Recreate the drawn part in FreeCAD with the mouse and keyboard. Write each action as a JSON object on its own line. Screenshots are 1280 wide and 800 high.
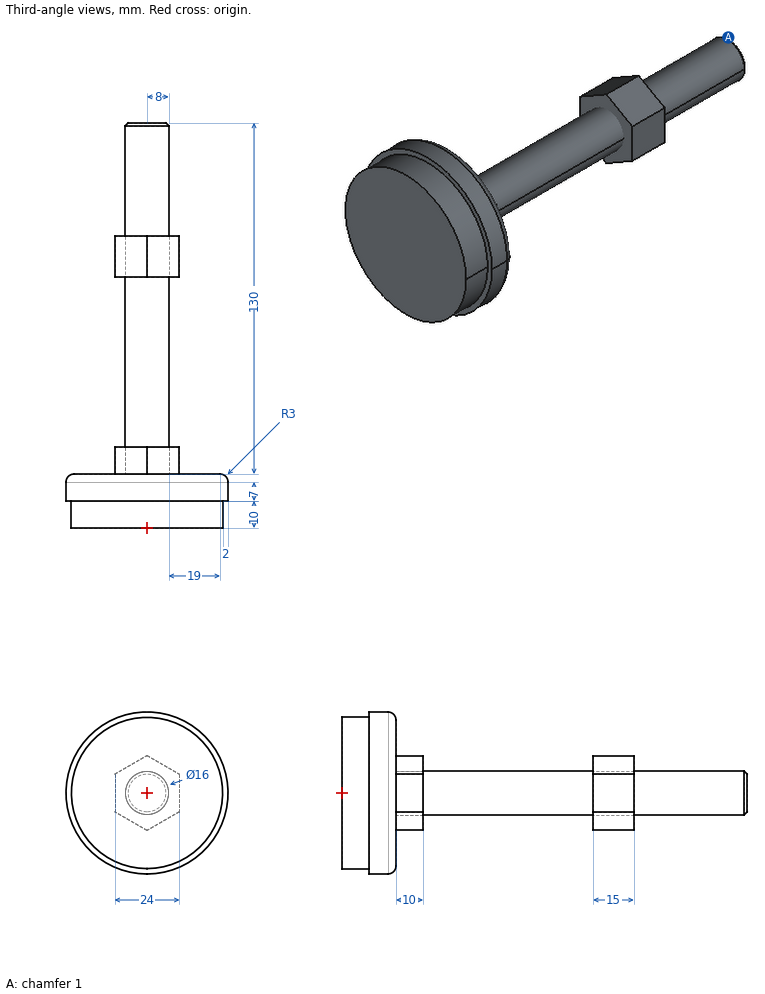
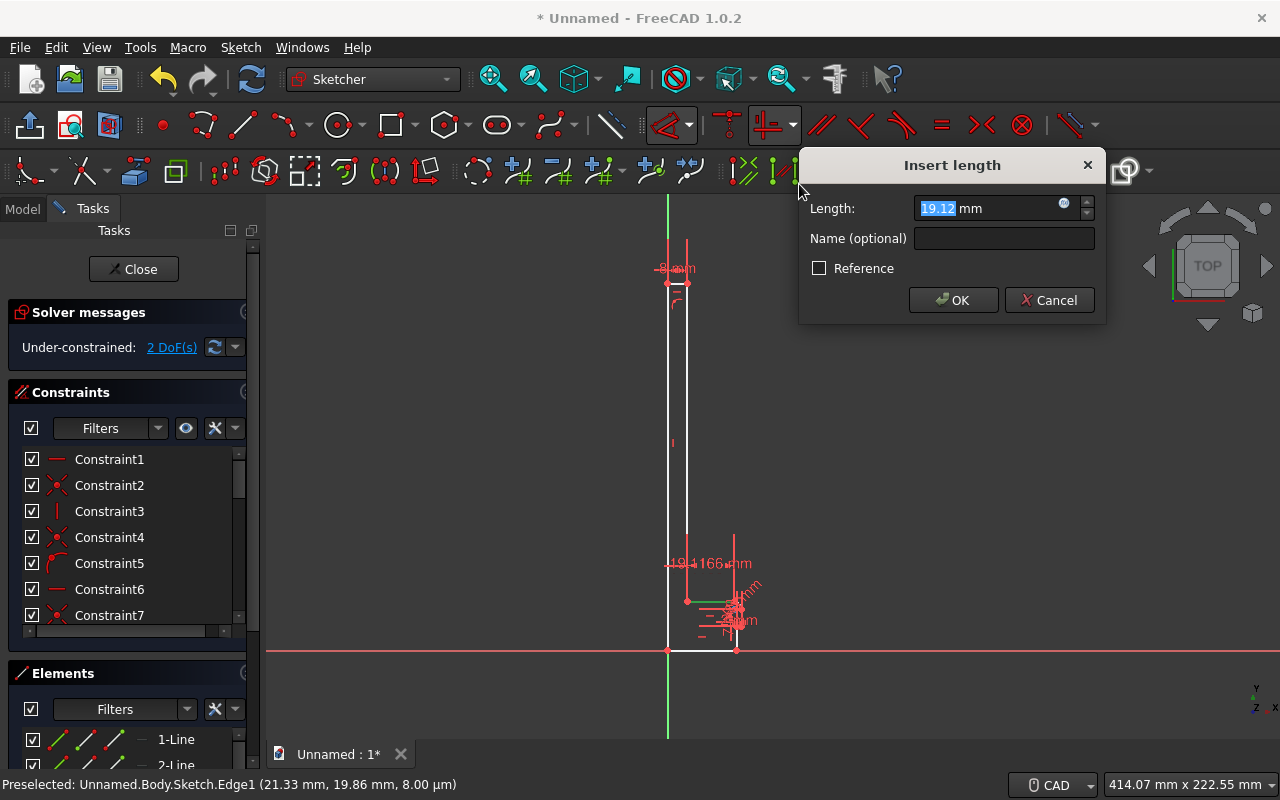
{"action": "type", "text": "19"}
{"action": "key", "text": "Return"}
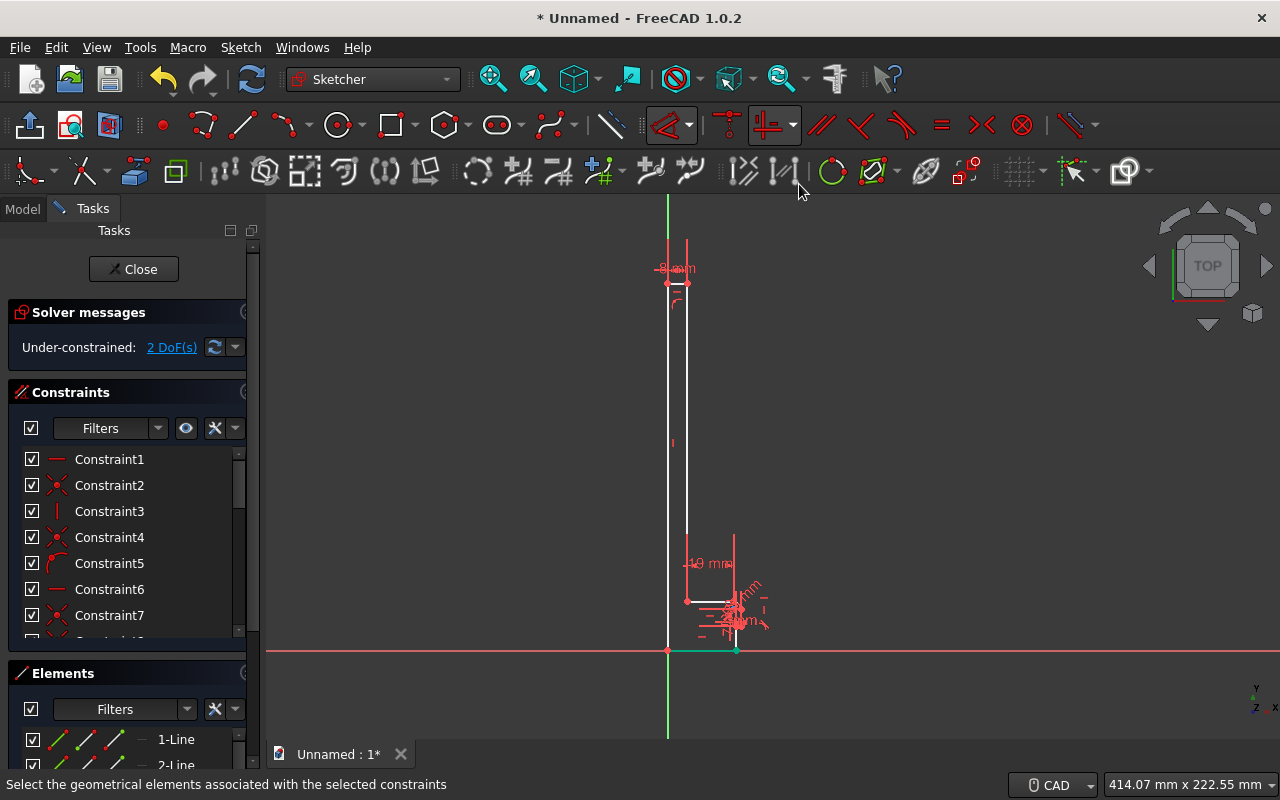
{"action": "scroll", "coordinate": [736, 641], "scroll_direction": "up", "scroll_amount": 3}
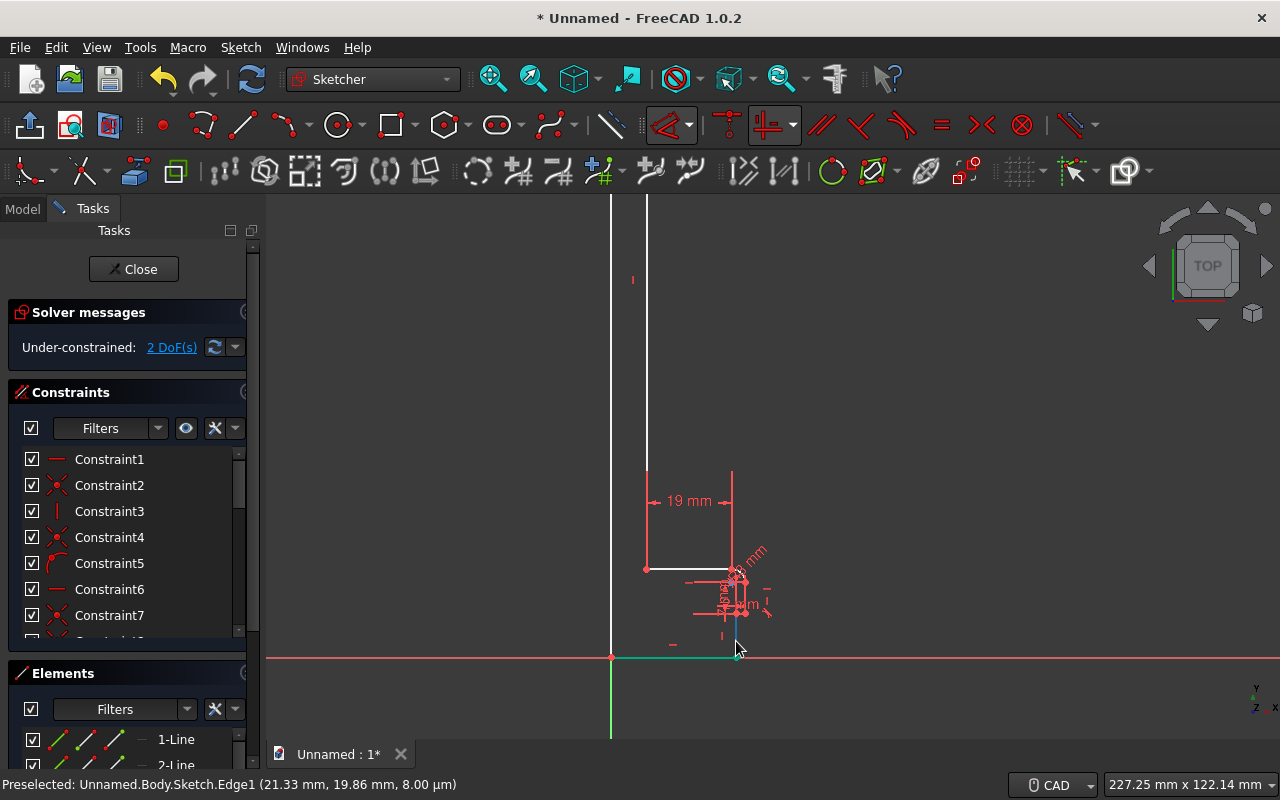
{"action": "left_click", "coordinate": [736, 640]}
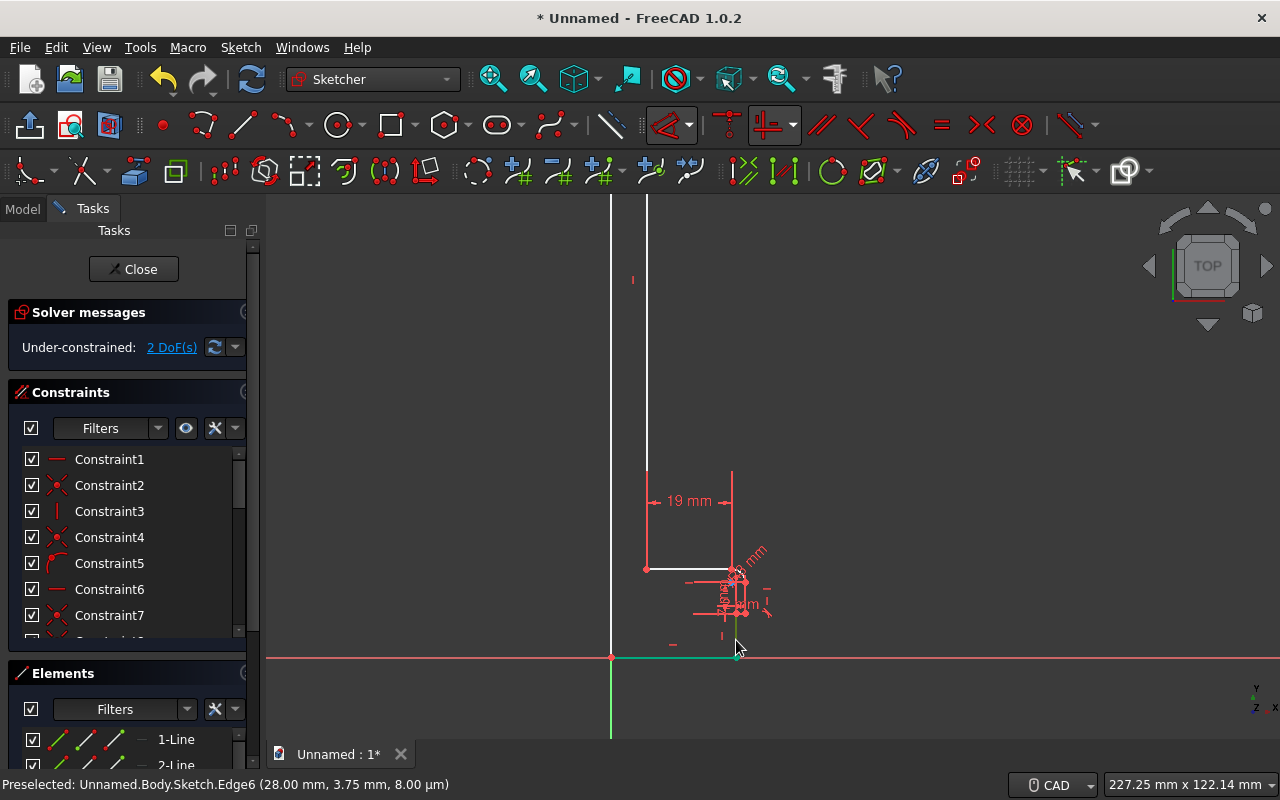
{"action": "key", "text": "i"}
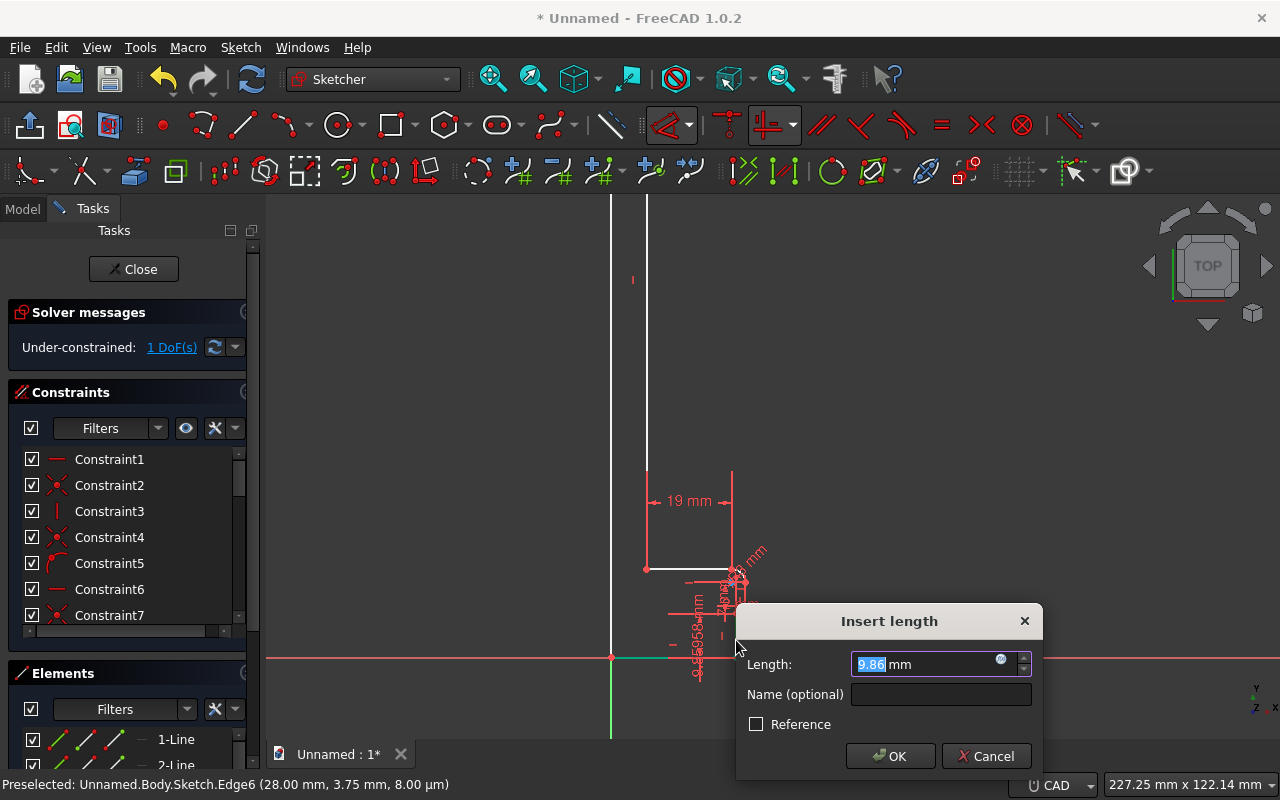
{"action": "type", "text": "10"}
{"action": "key", "text": "Return"}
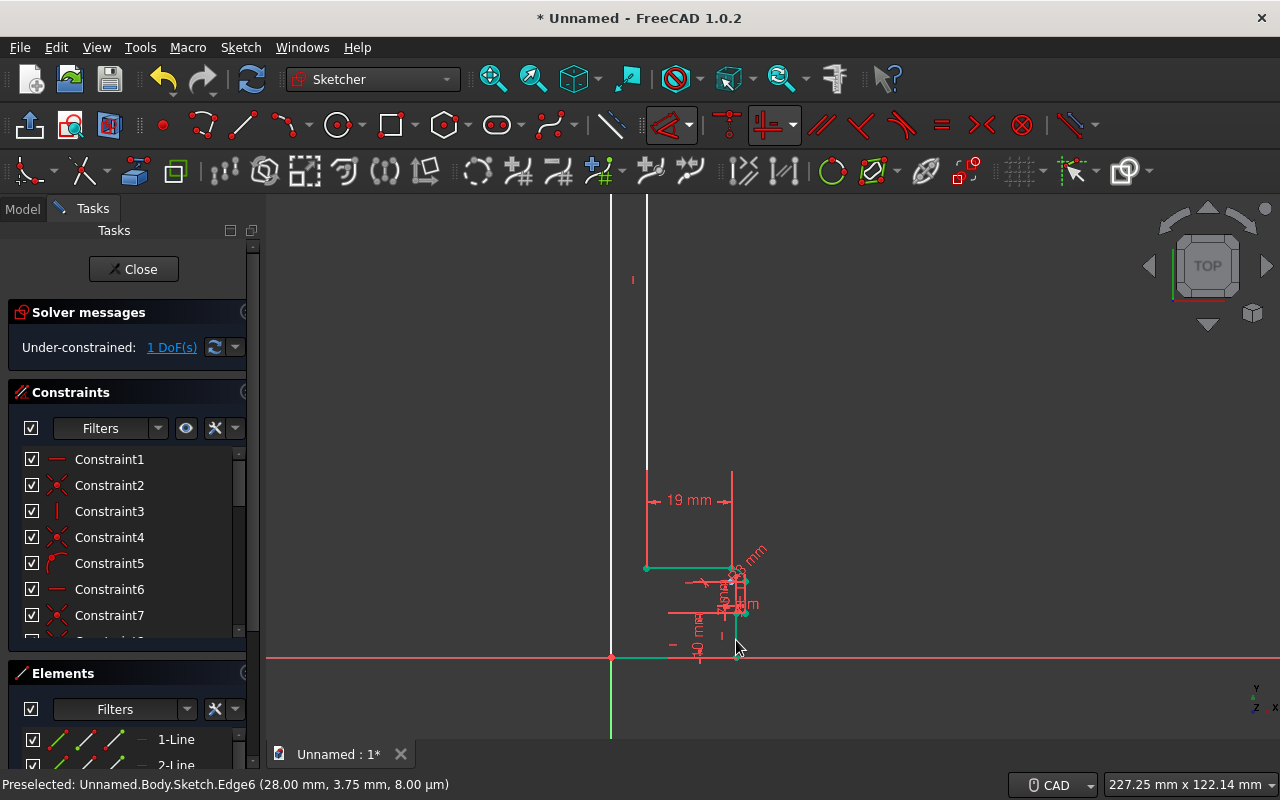
{"action": "left_click", "coordinate": [647, 395]}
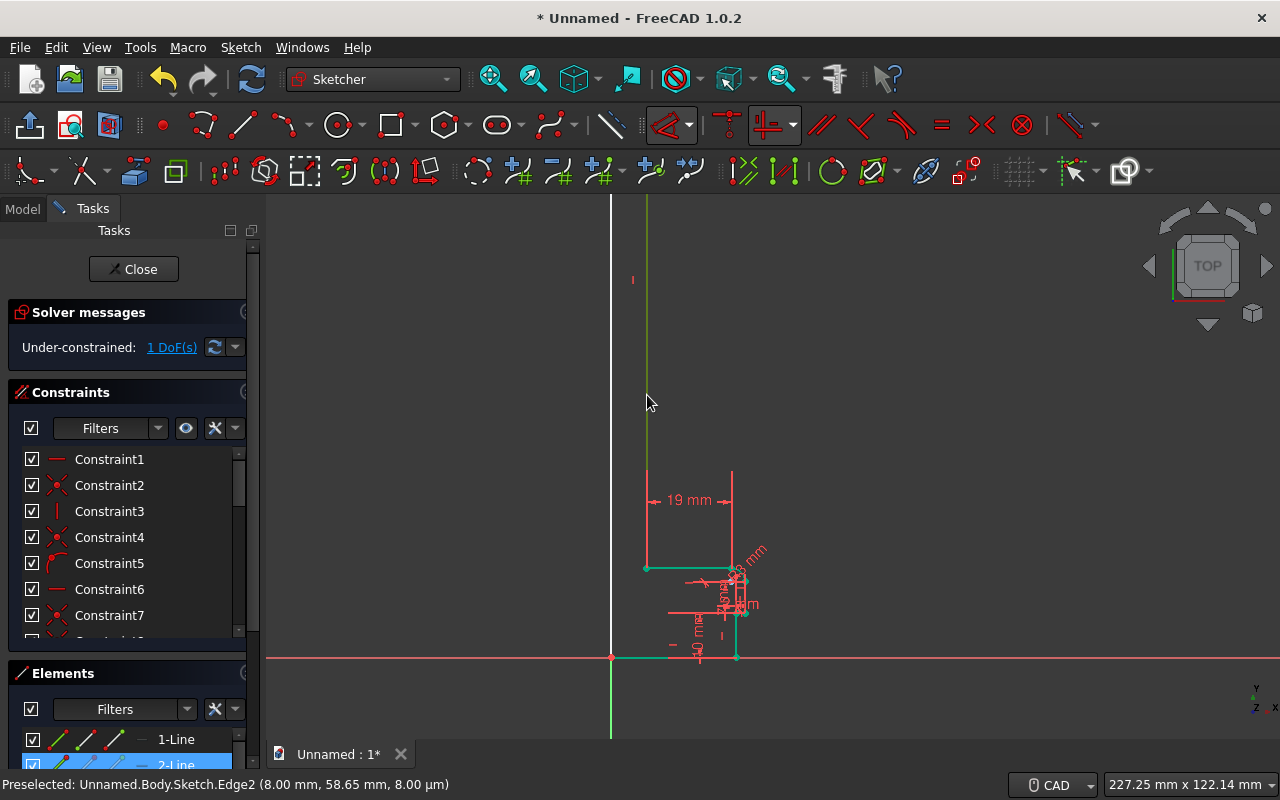
{"action": "left_click", "coordinate": [692, 126]}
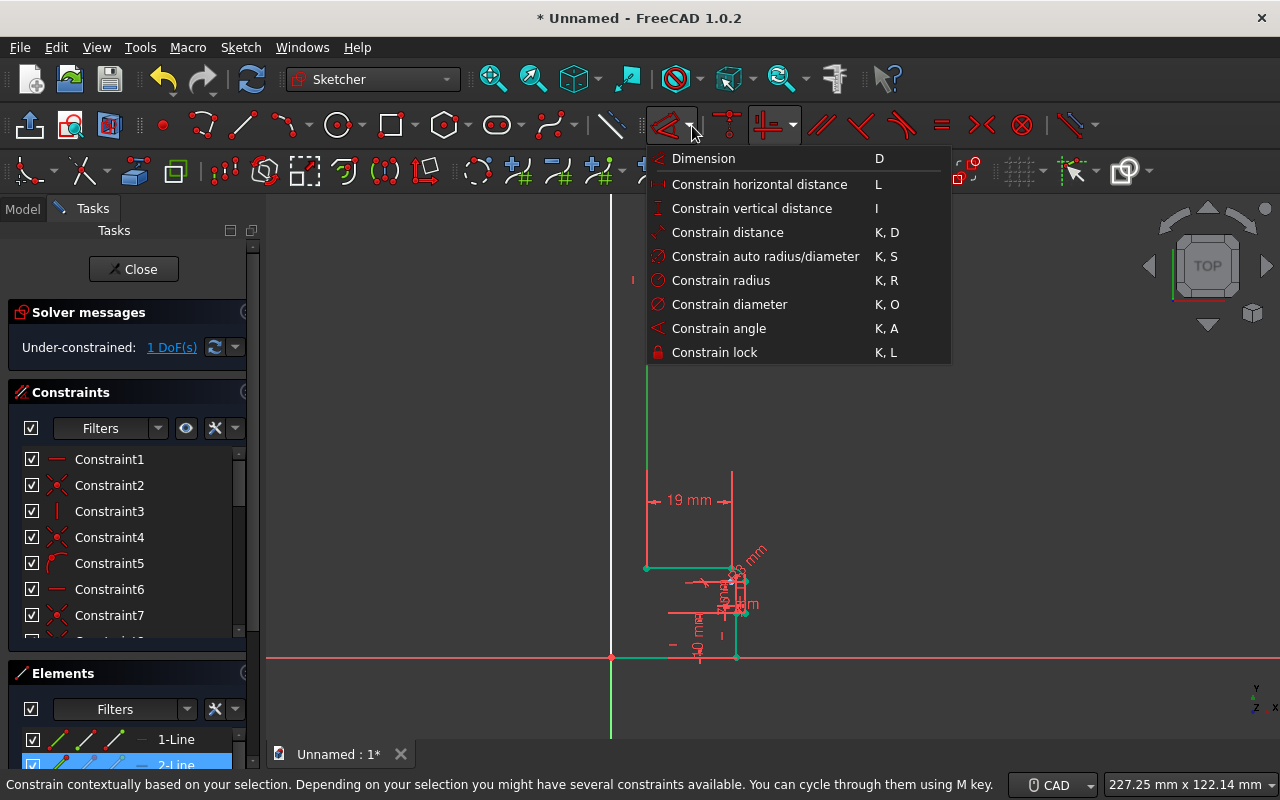
{"action": "left_click", "coordinate": [799, 208]}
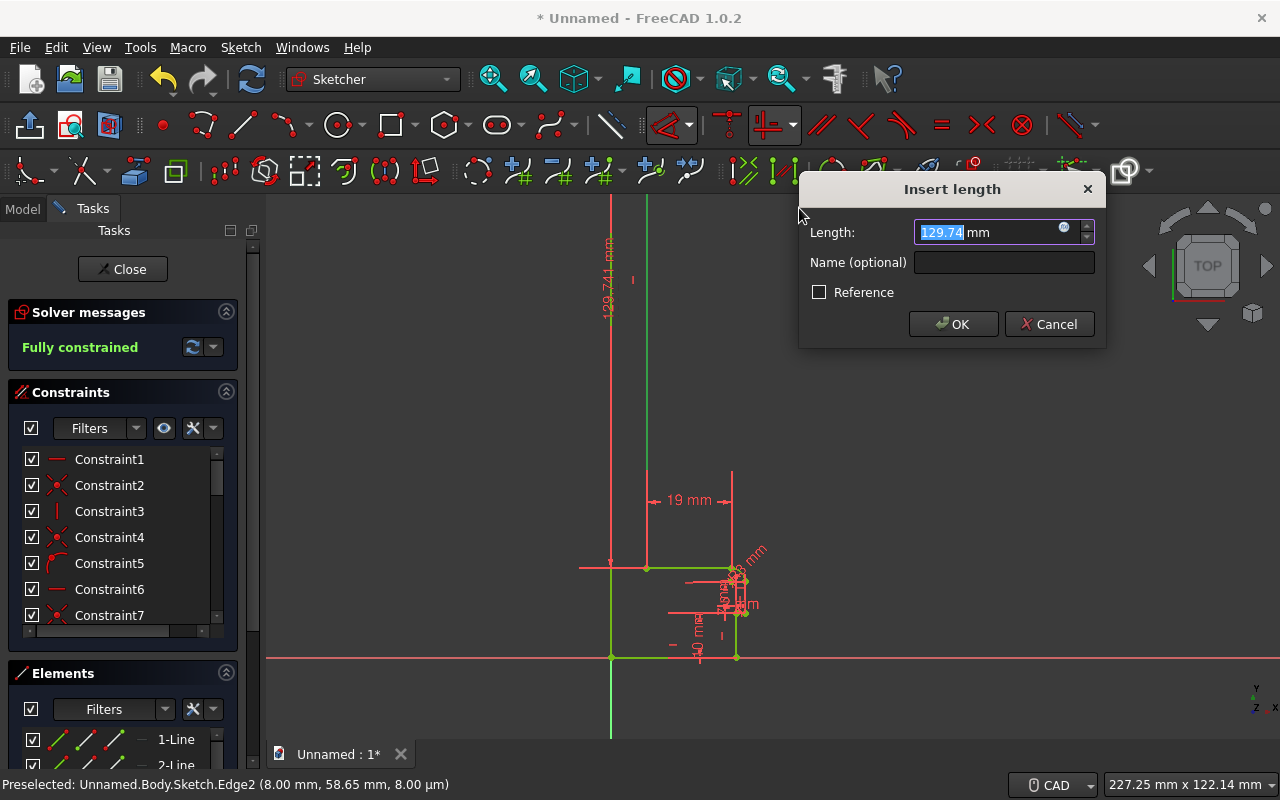
{"action": "type", "text": "130"}
{"action": "key", "text": "Return"}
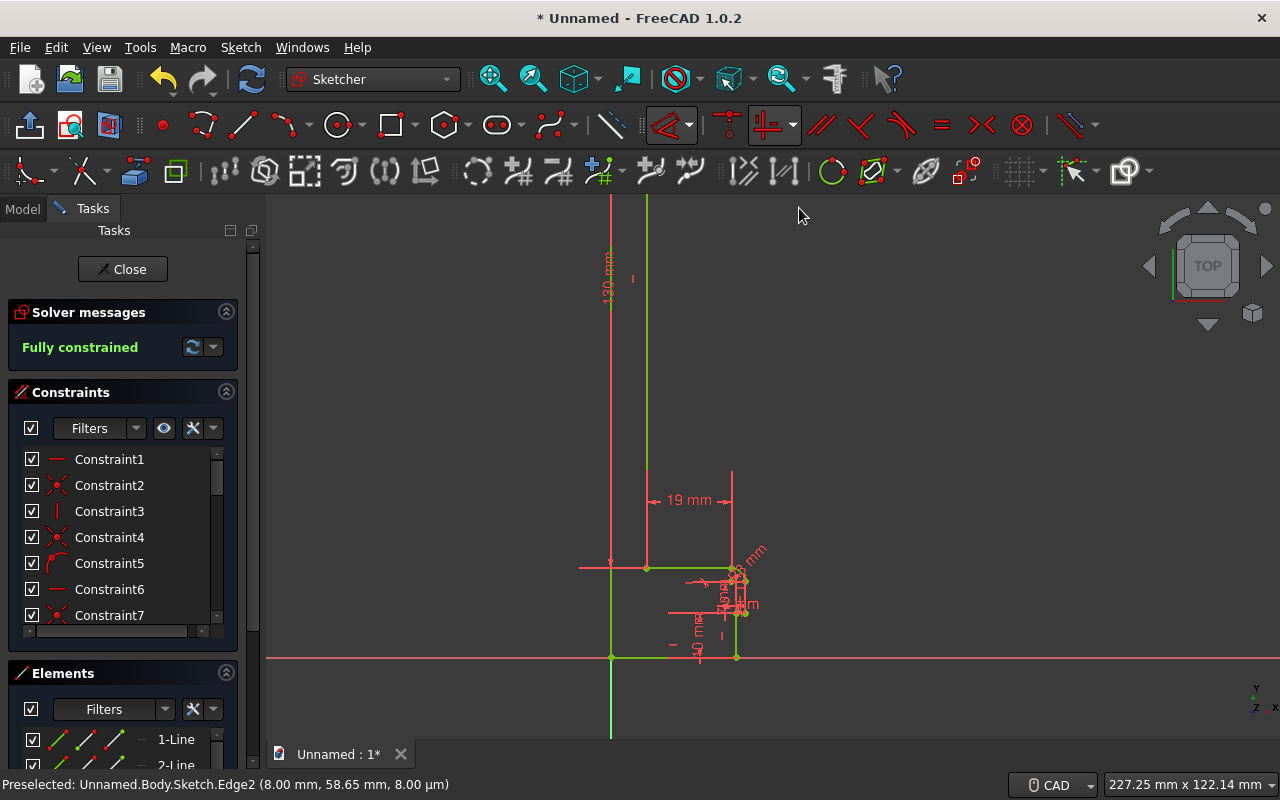
{"action": "left_click", "coordinate": [123, 269]}